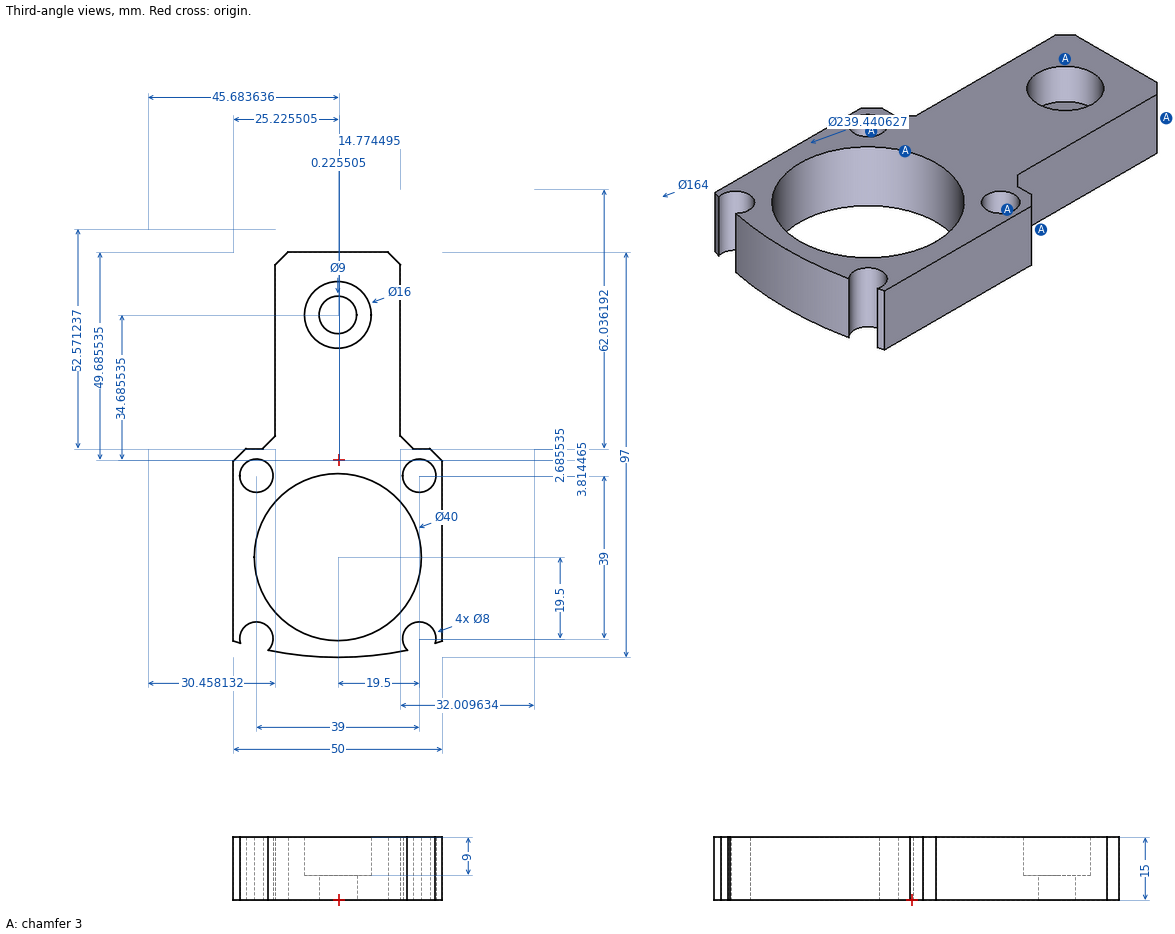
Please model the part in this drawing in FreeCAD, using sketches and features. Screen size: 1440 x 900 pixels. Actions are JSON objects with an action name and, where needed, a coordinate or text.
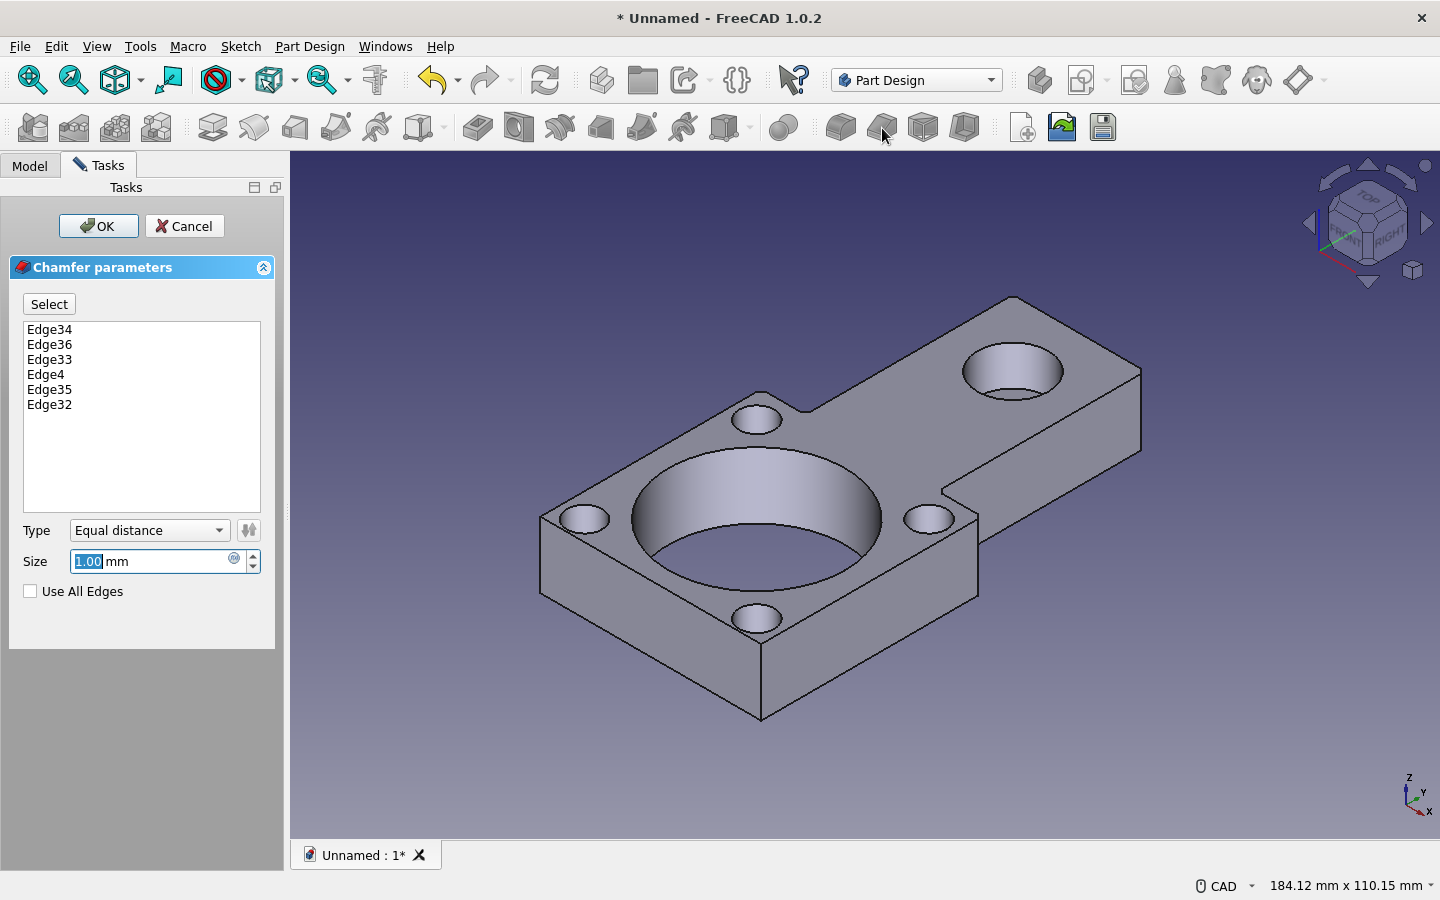
{"action": "type", "text": "3"}
{"action": "key", "text": "Tab"}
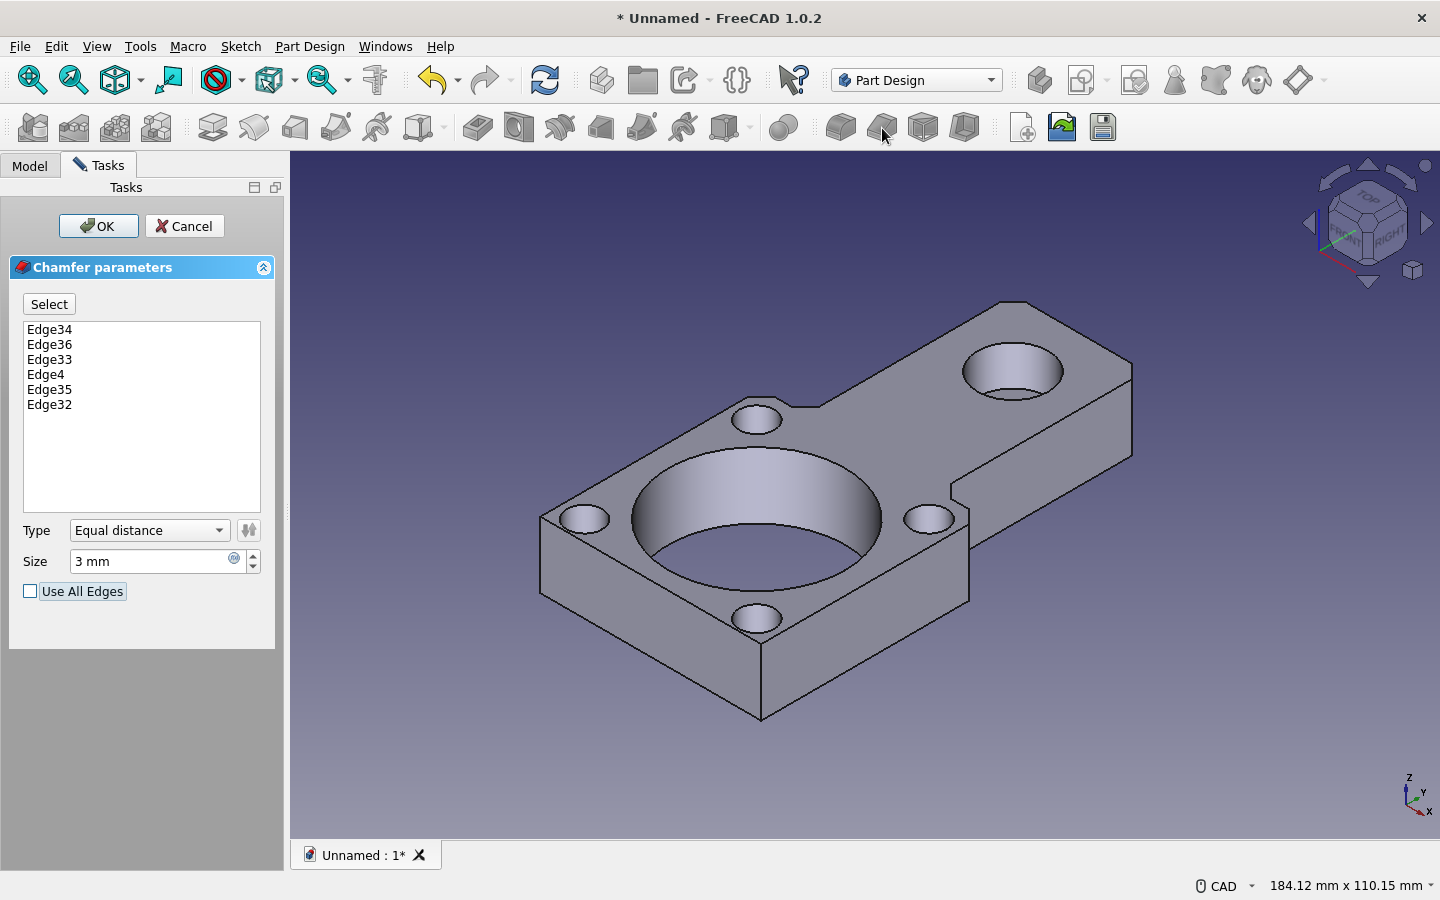
{"action": "left_click", "coordinate": [99, 226]}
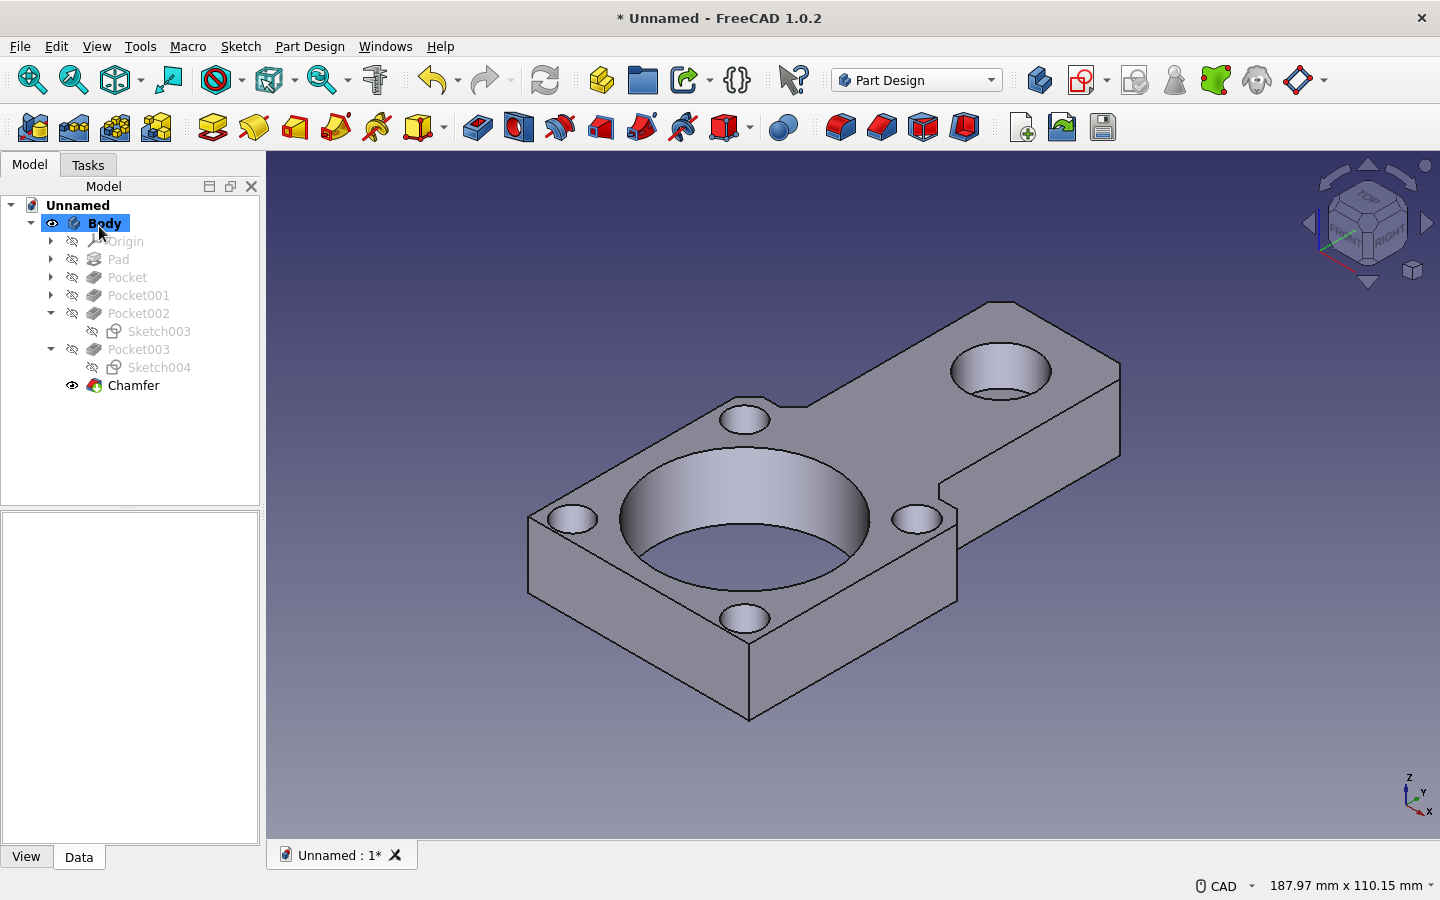
{"action": "key", "text": "5"}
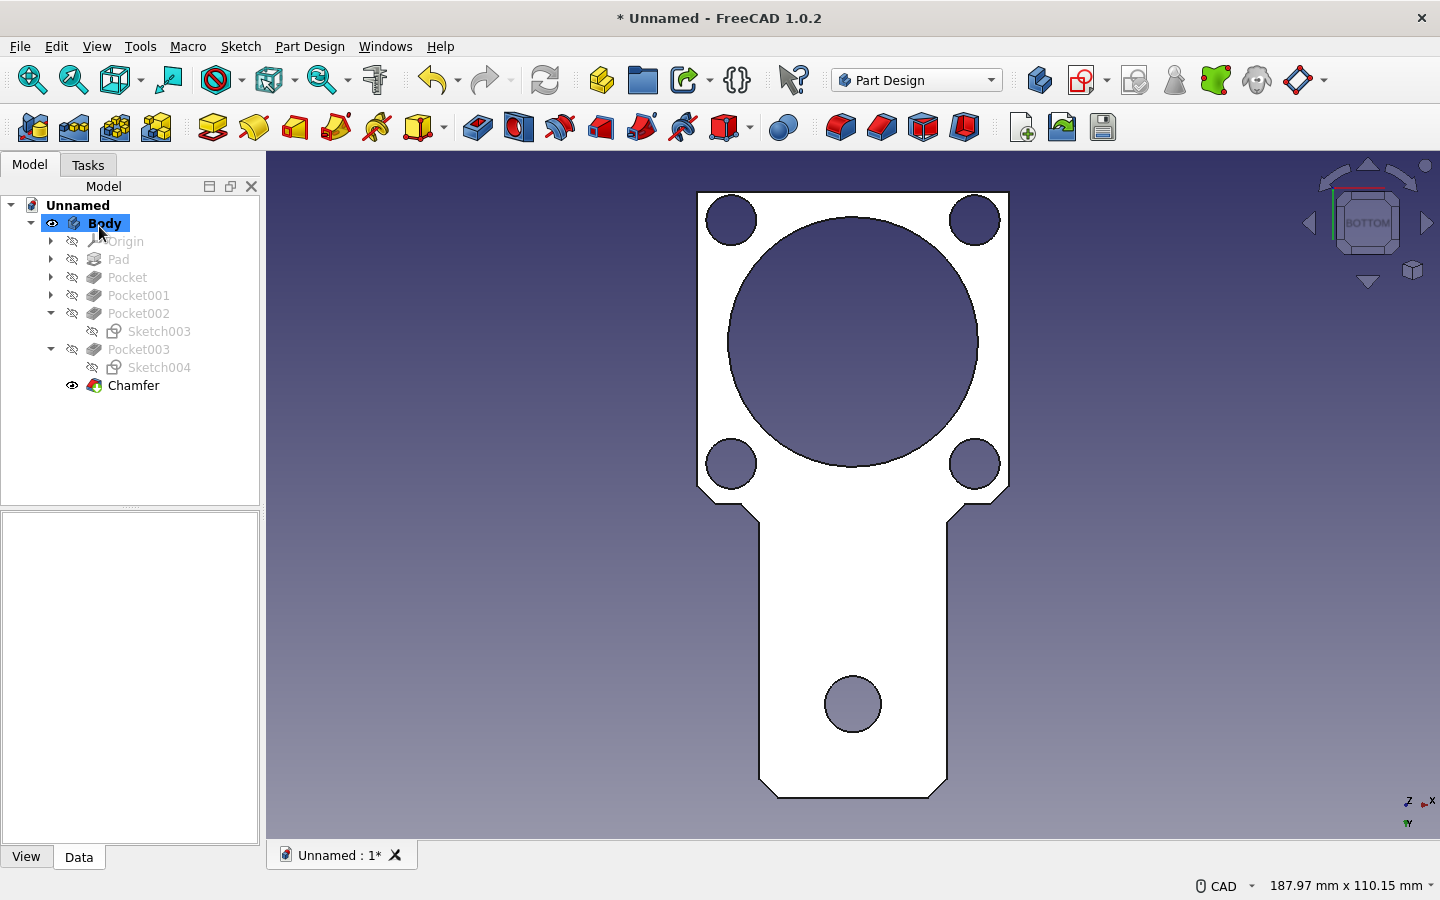
{"action": "left_click", "coordinate": [853, 581]}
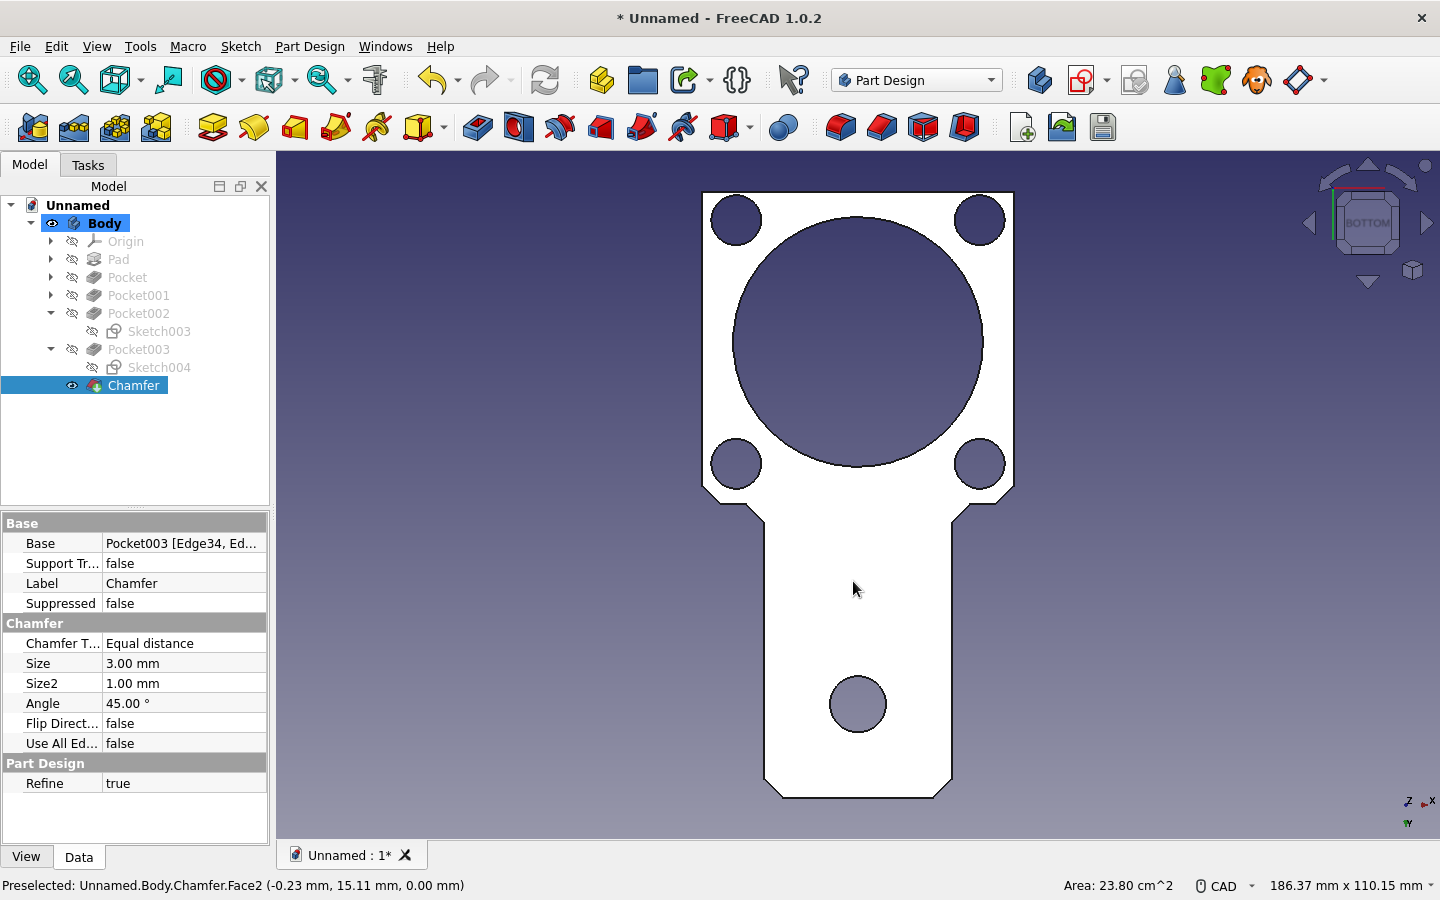
{"action": "left_click", "coordinate": [1080, 80]}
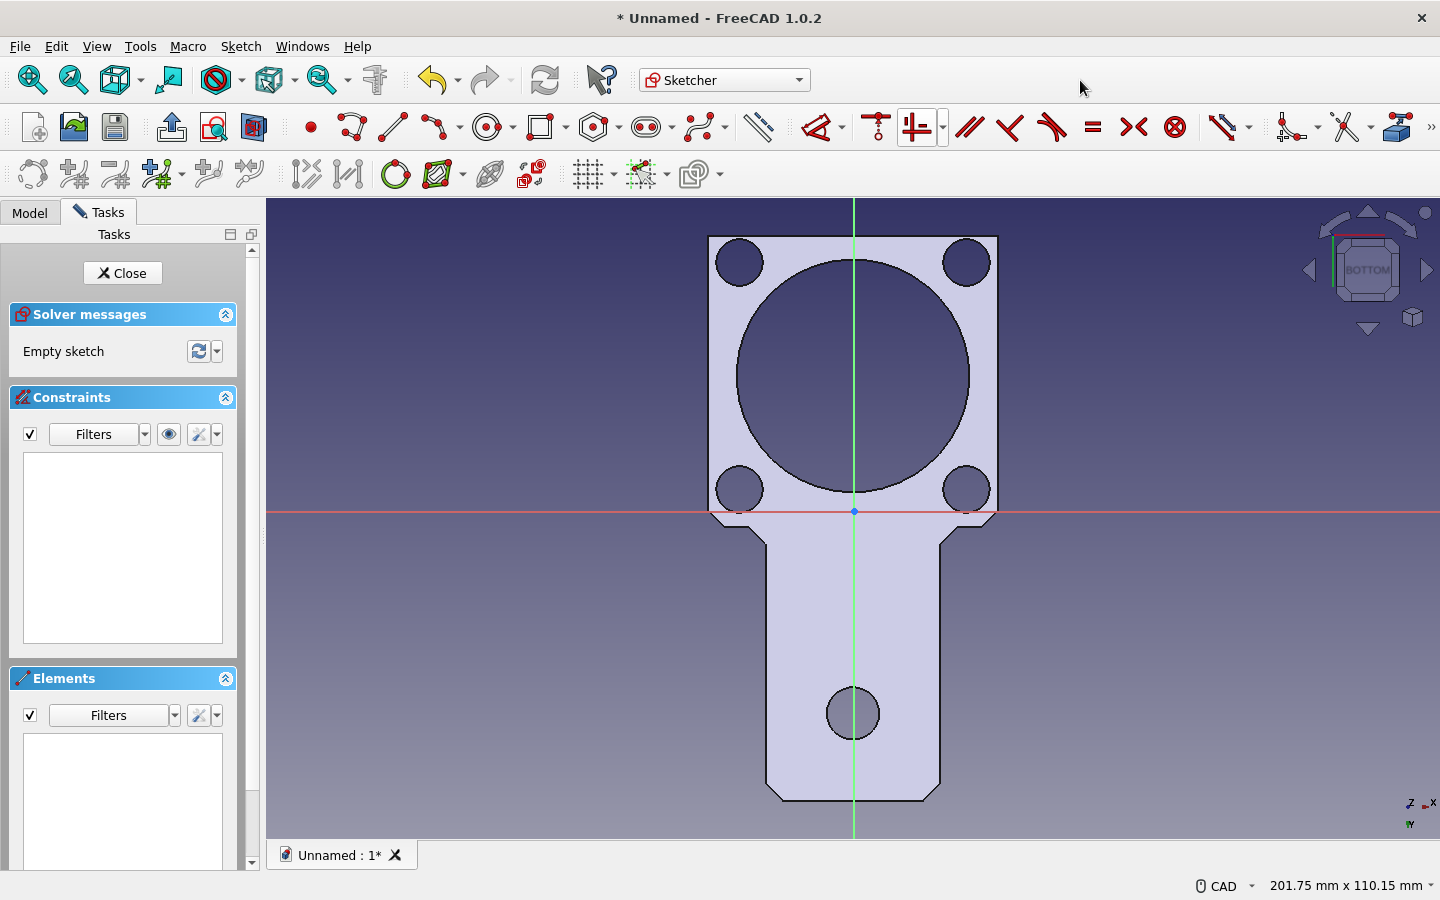
{"action": "scroll", "coordinate": [755, 434], "scroll_direction": "down", "scroll_amount": 6}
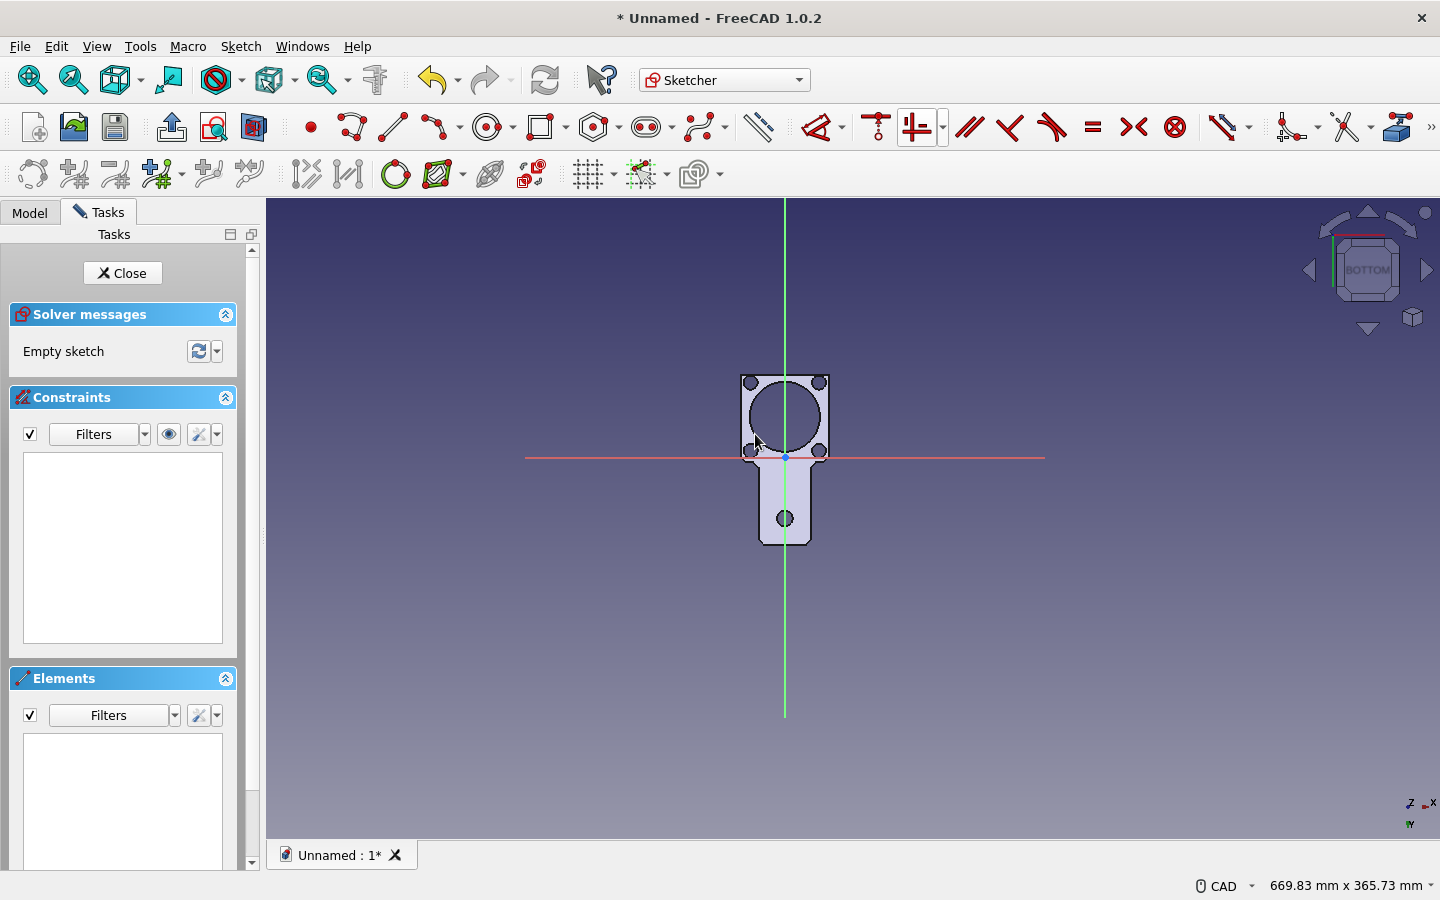
{"action": "left_click", "coordinate": [486, 128]}